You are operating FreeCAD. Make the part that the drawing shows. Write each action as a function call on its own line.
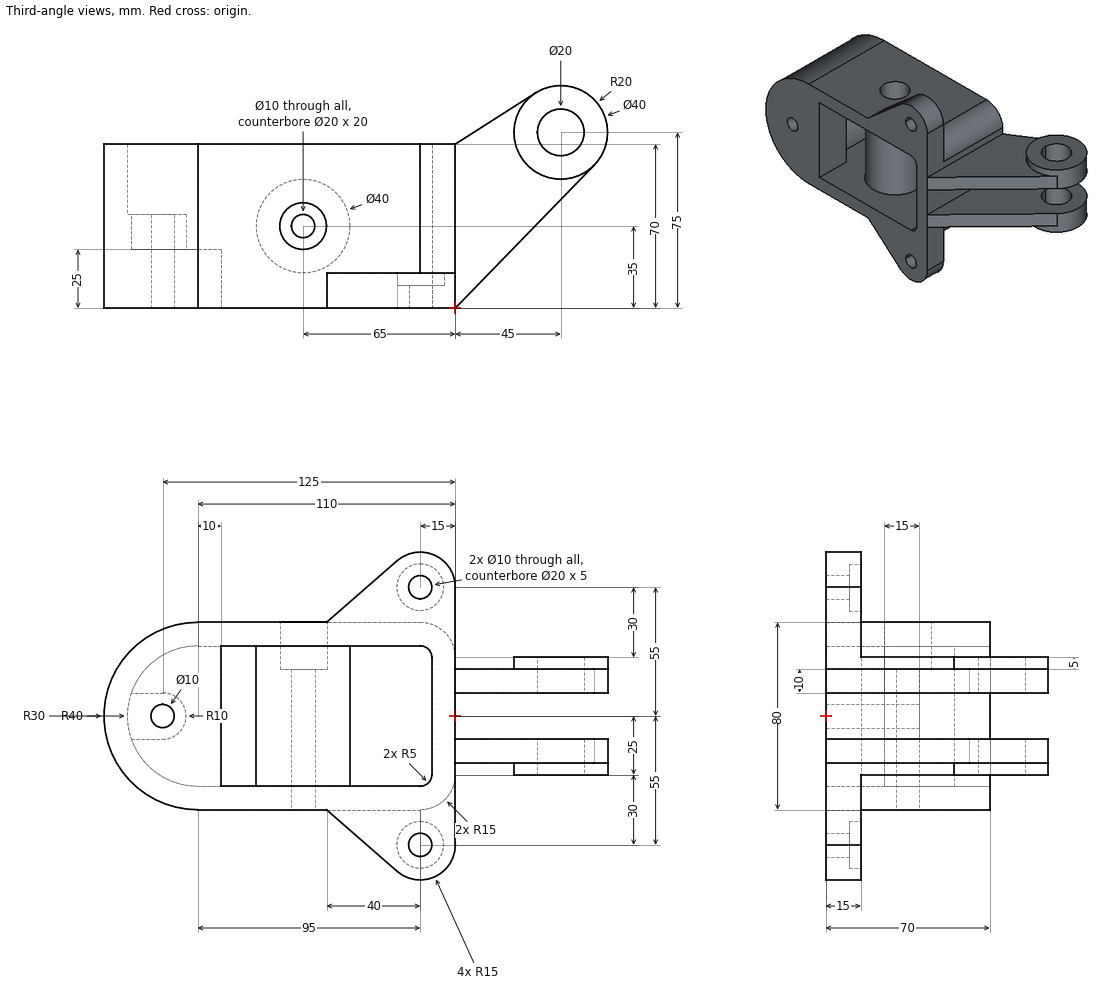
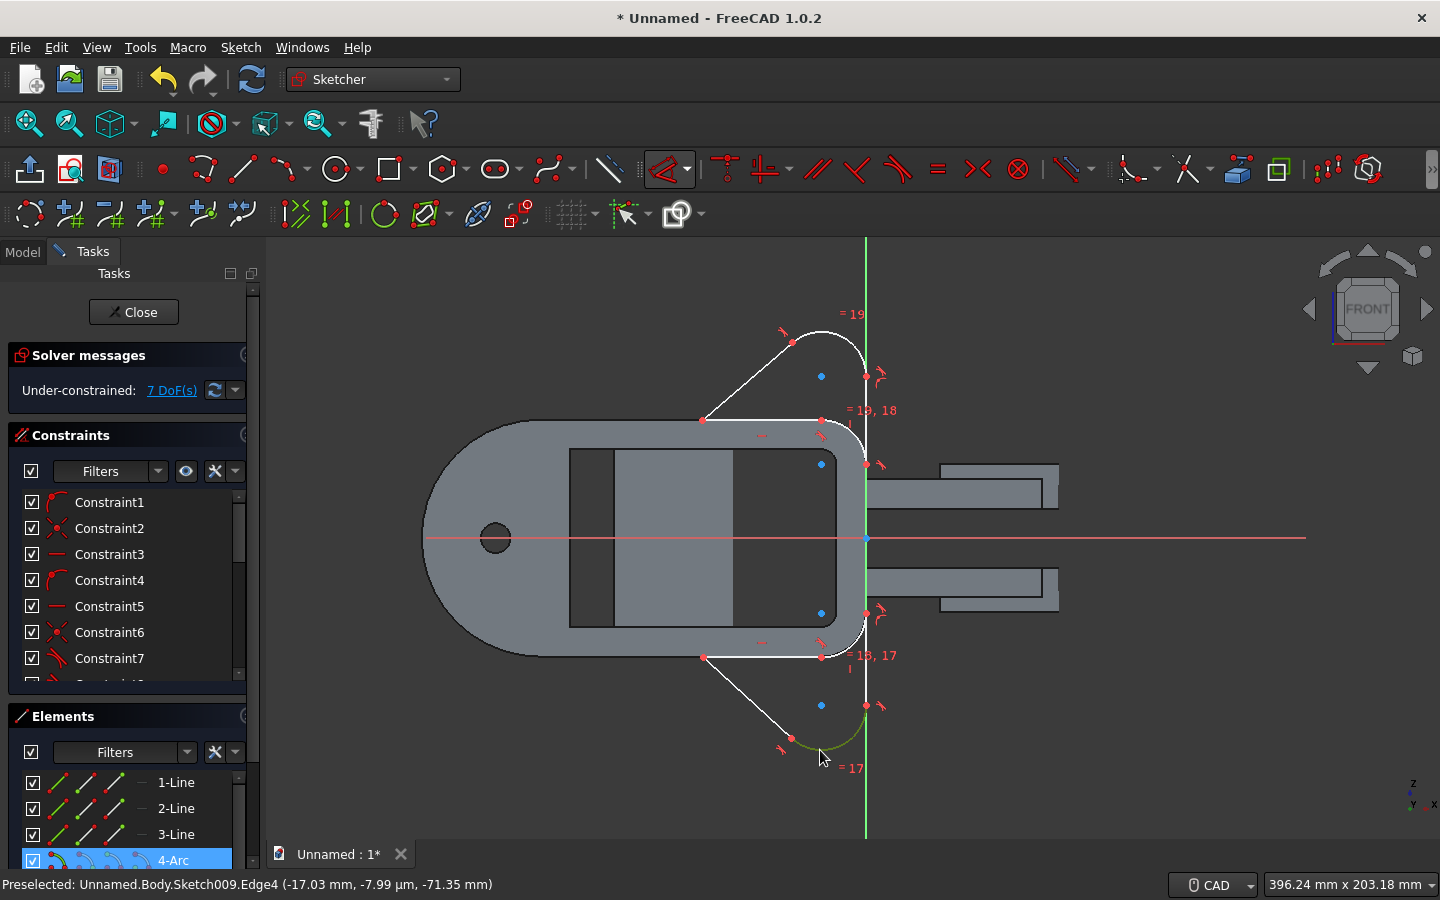
key(k)
key(r)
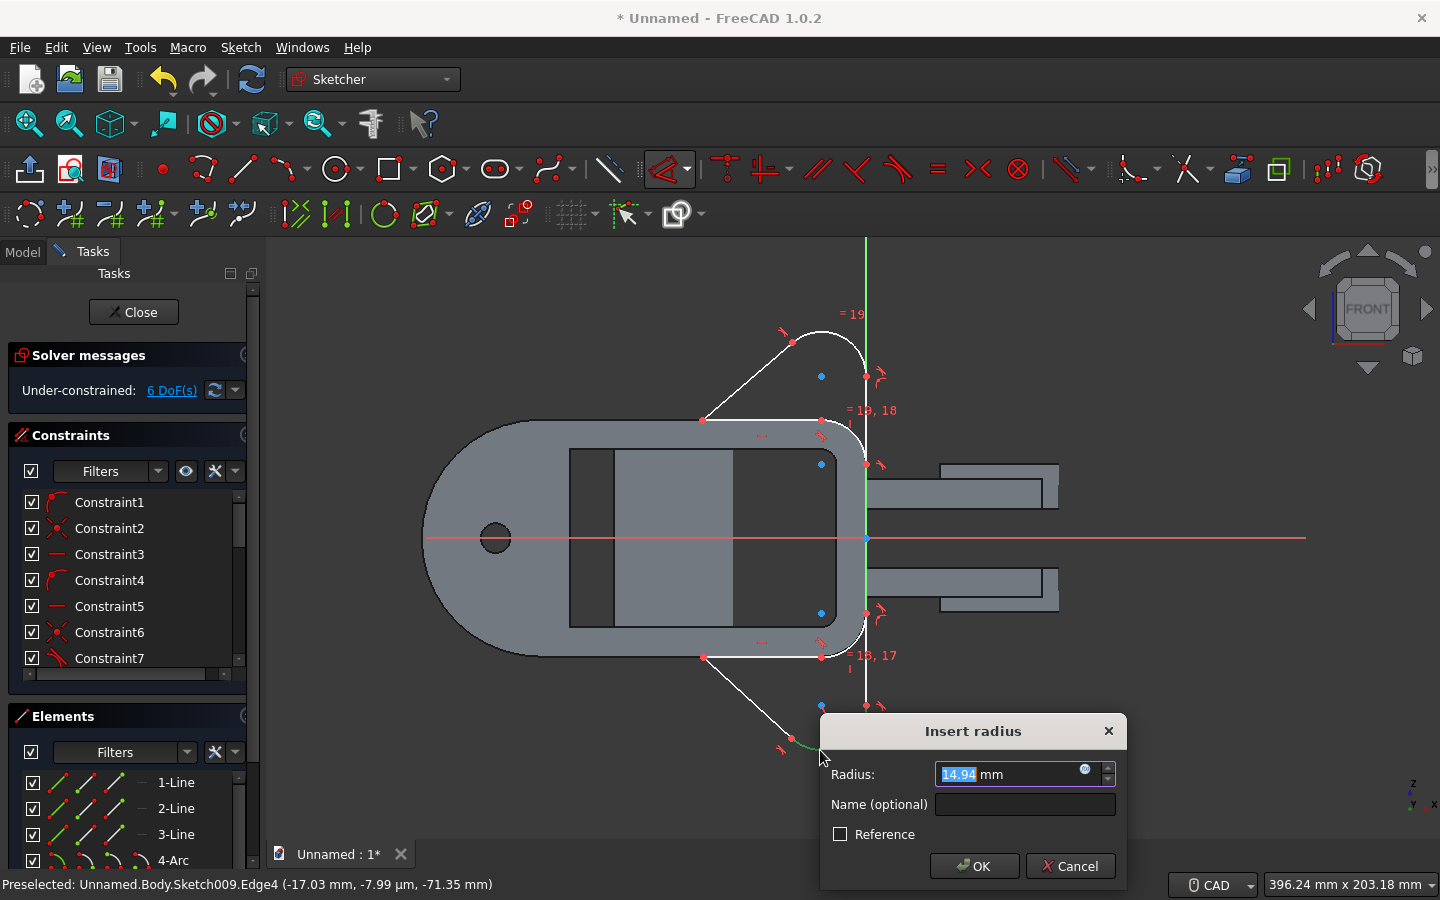
text(15)
key(Return)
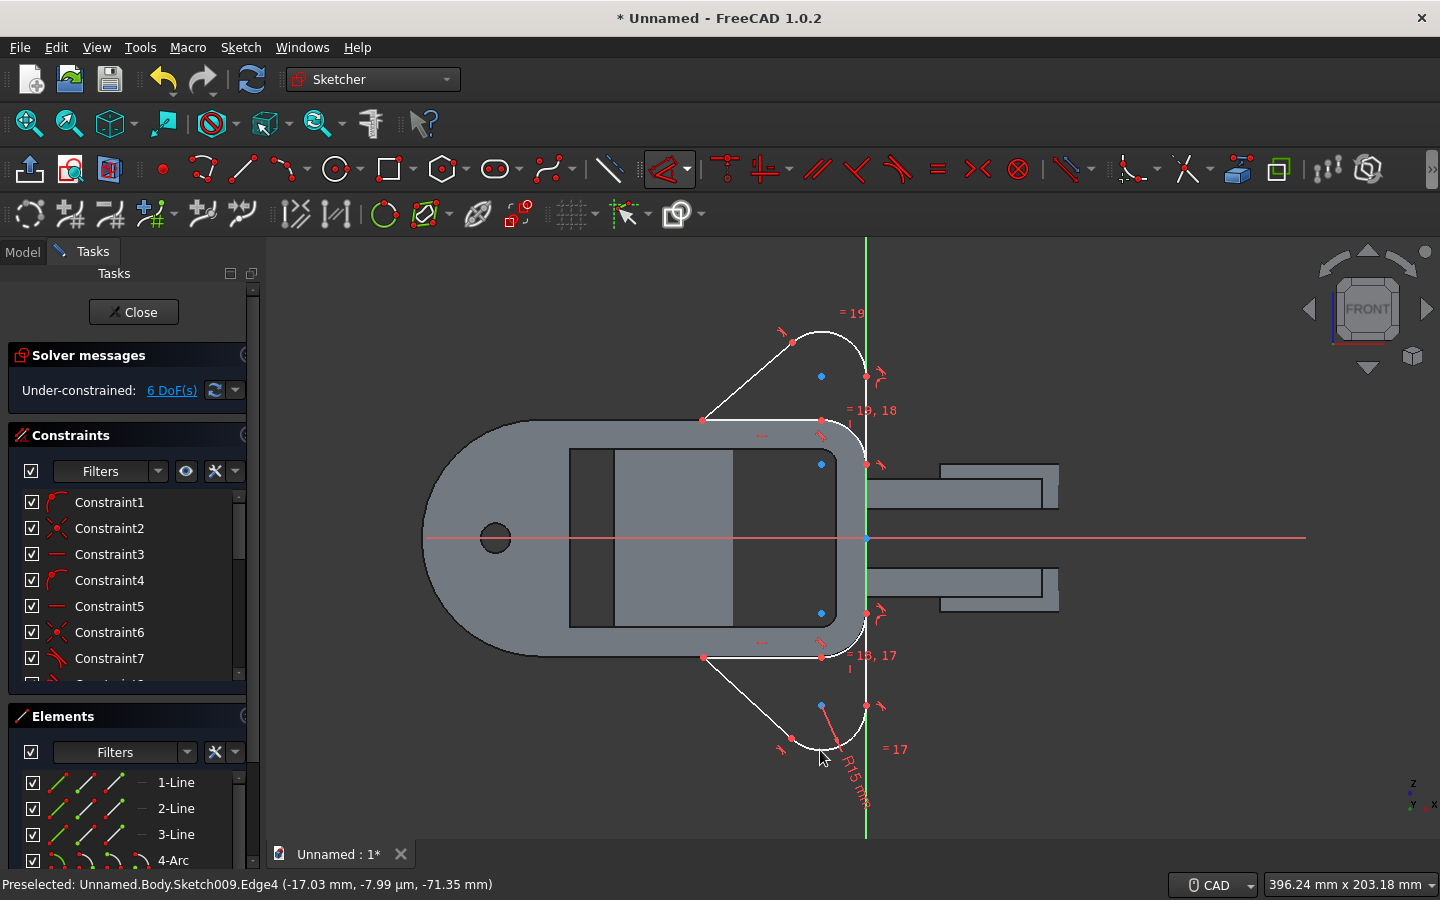
click(866, 678)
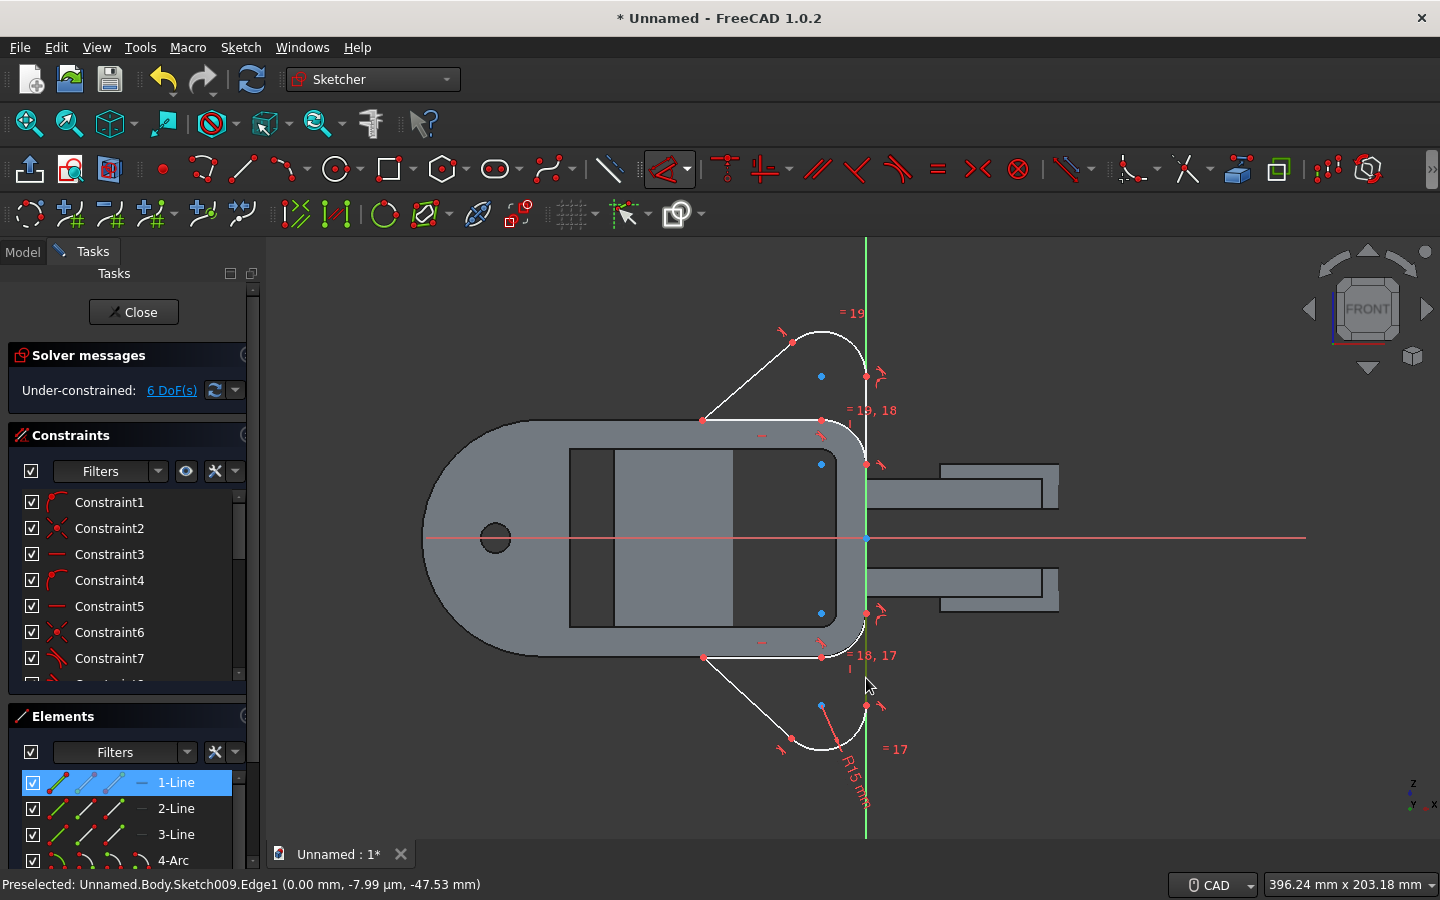
key(i)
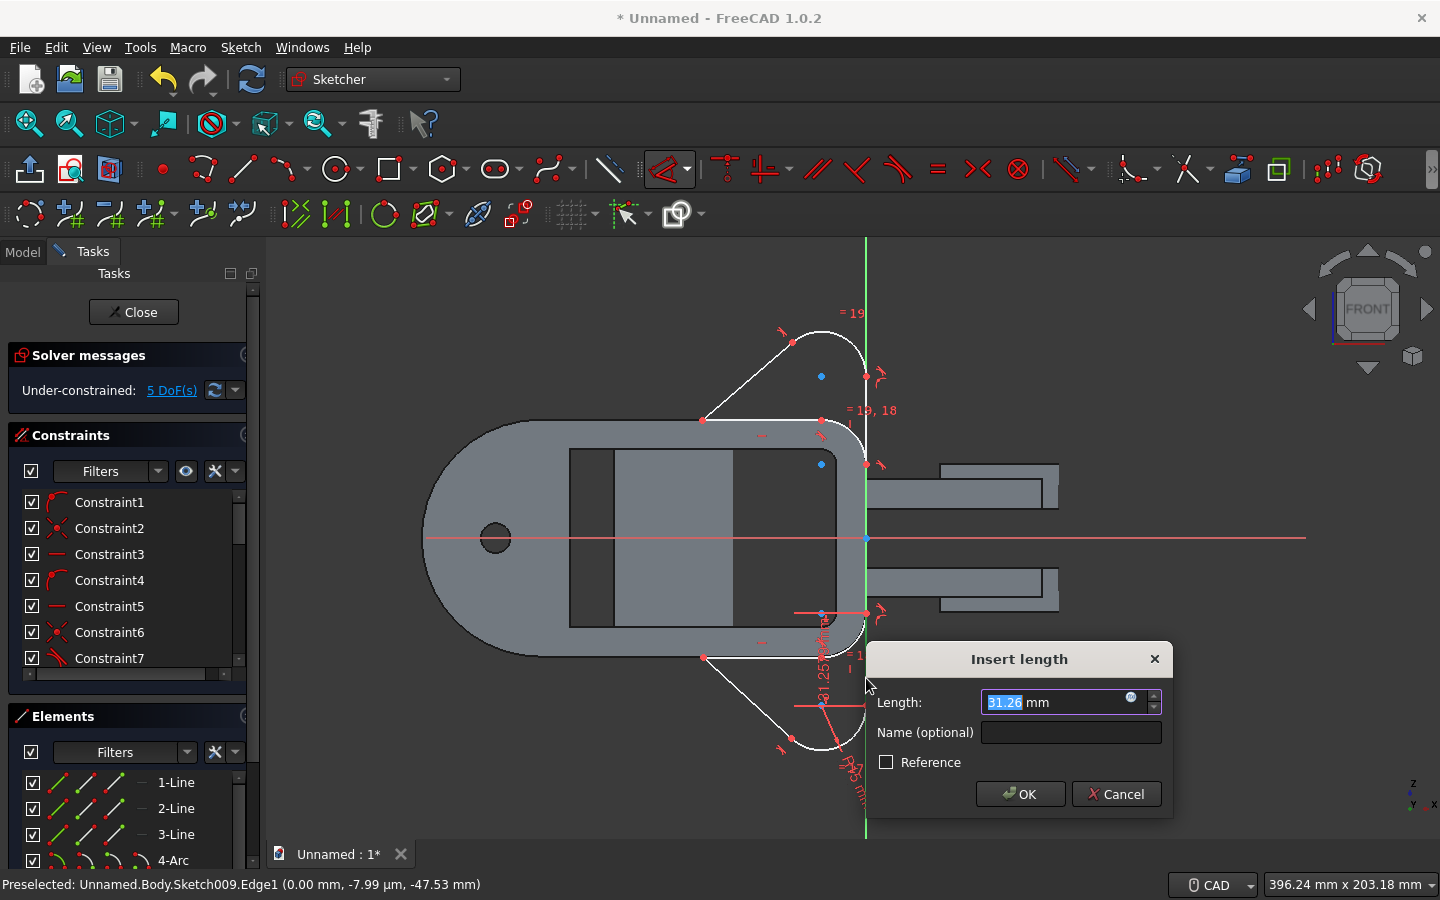
text(30)
key(Return)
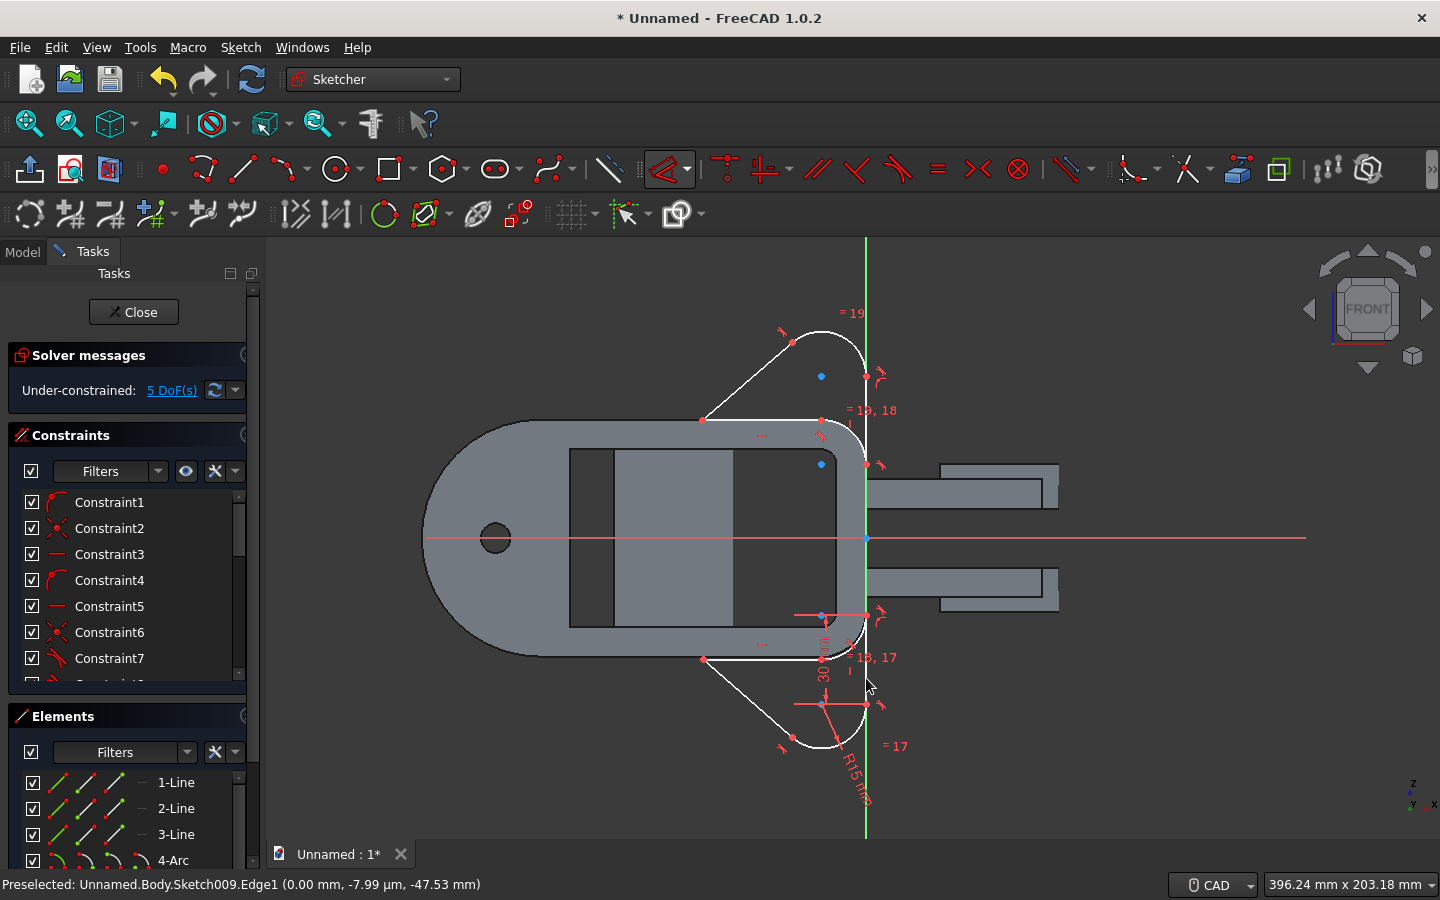
click(739, 660)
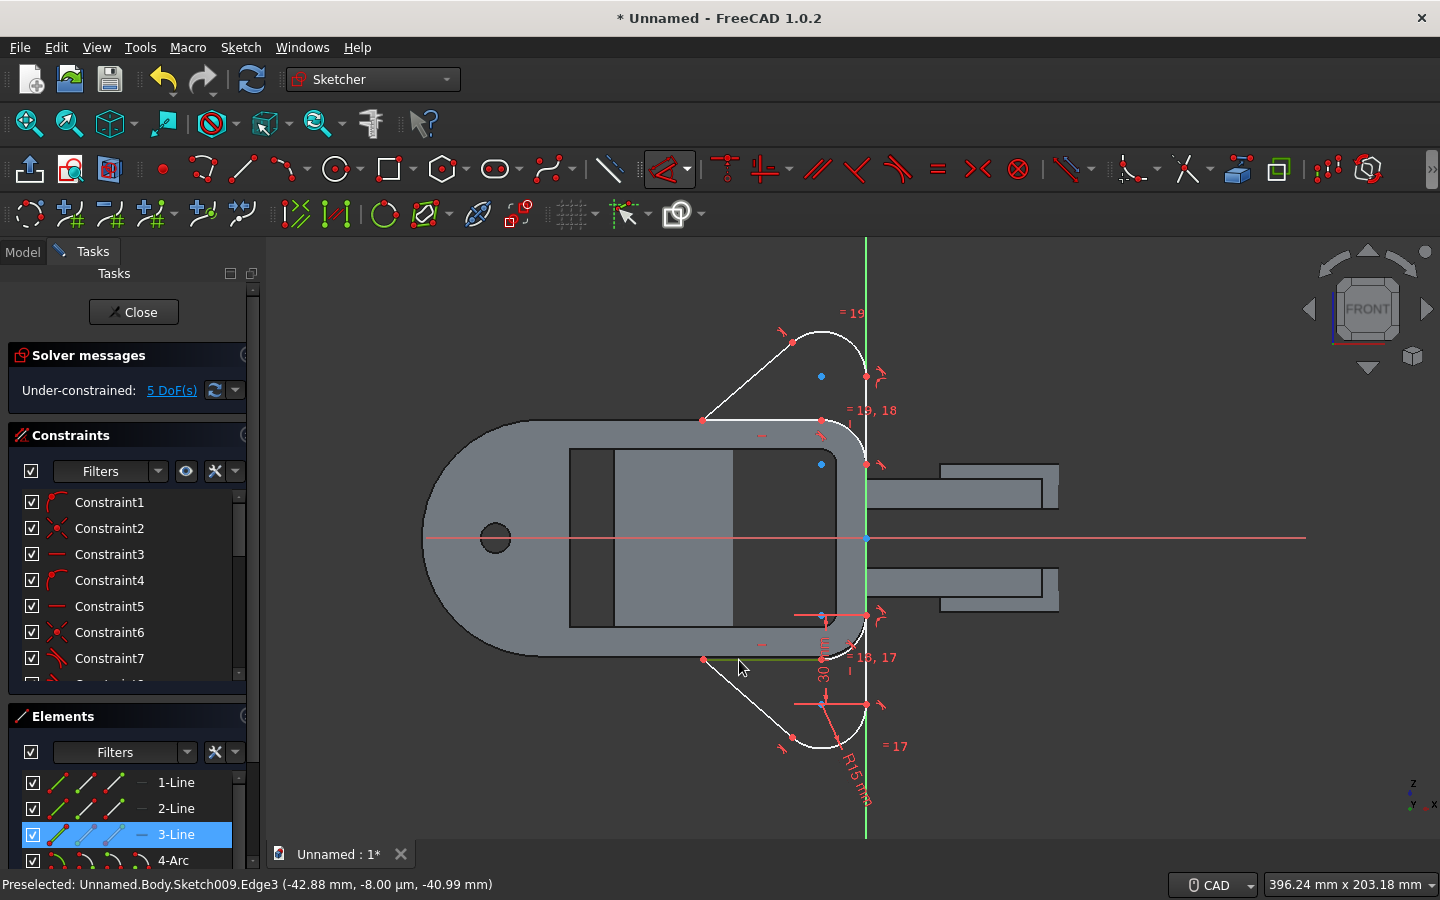
key(l)